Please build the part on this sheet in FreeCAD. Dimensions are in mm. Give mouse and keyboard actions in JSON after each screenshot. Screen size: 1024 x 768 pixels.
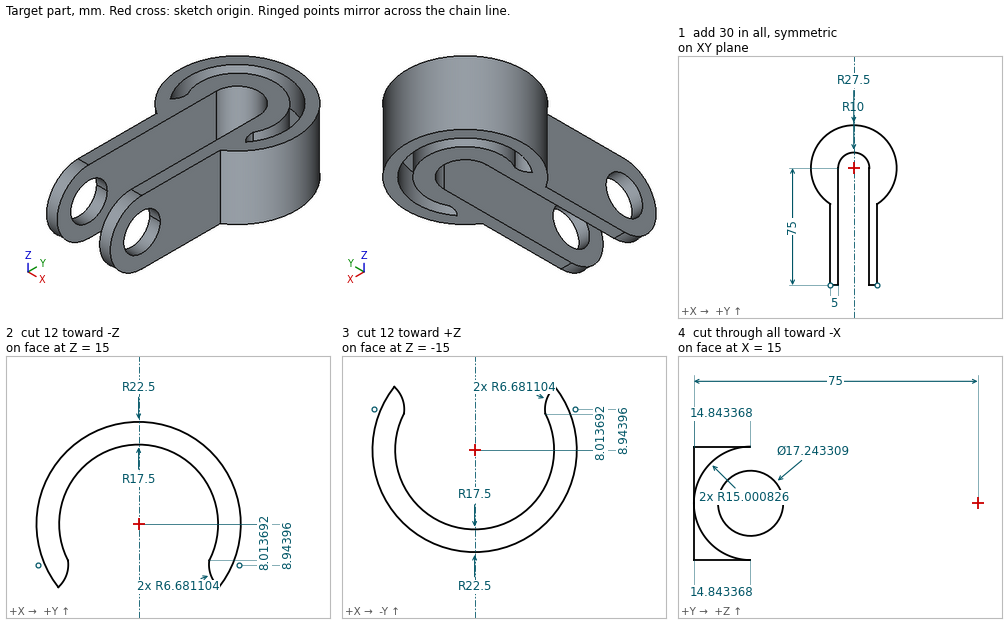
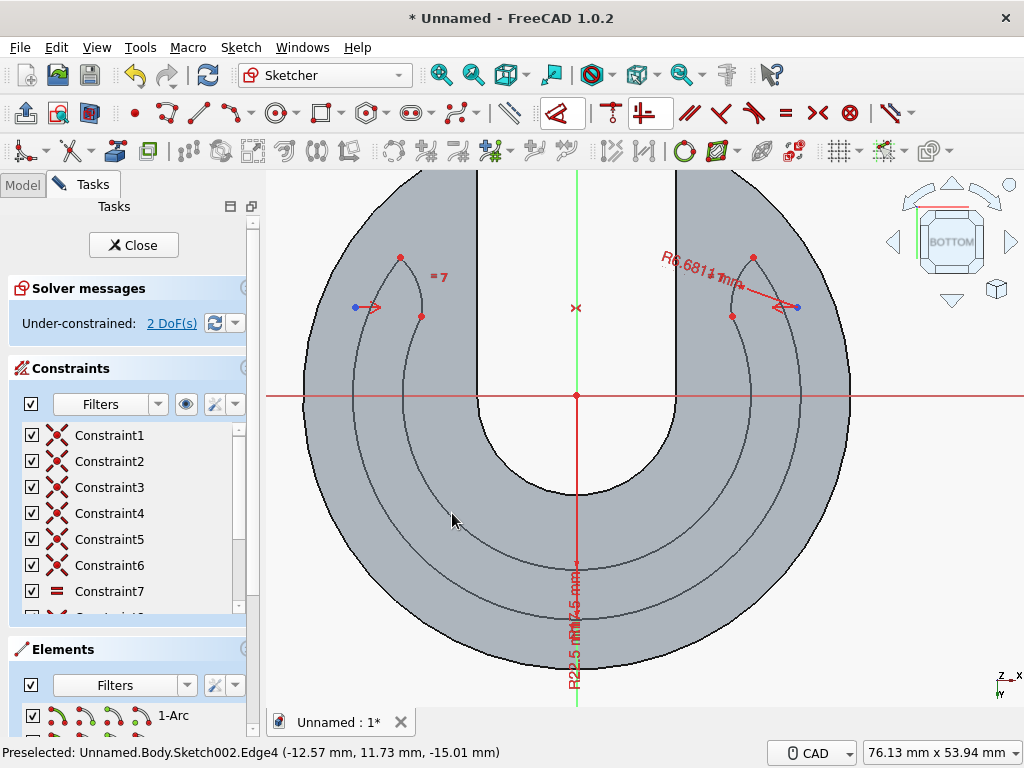
{"action": "left_click", "coordinate": [798, 307]}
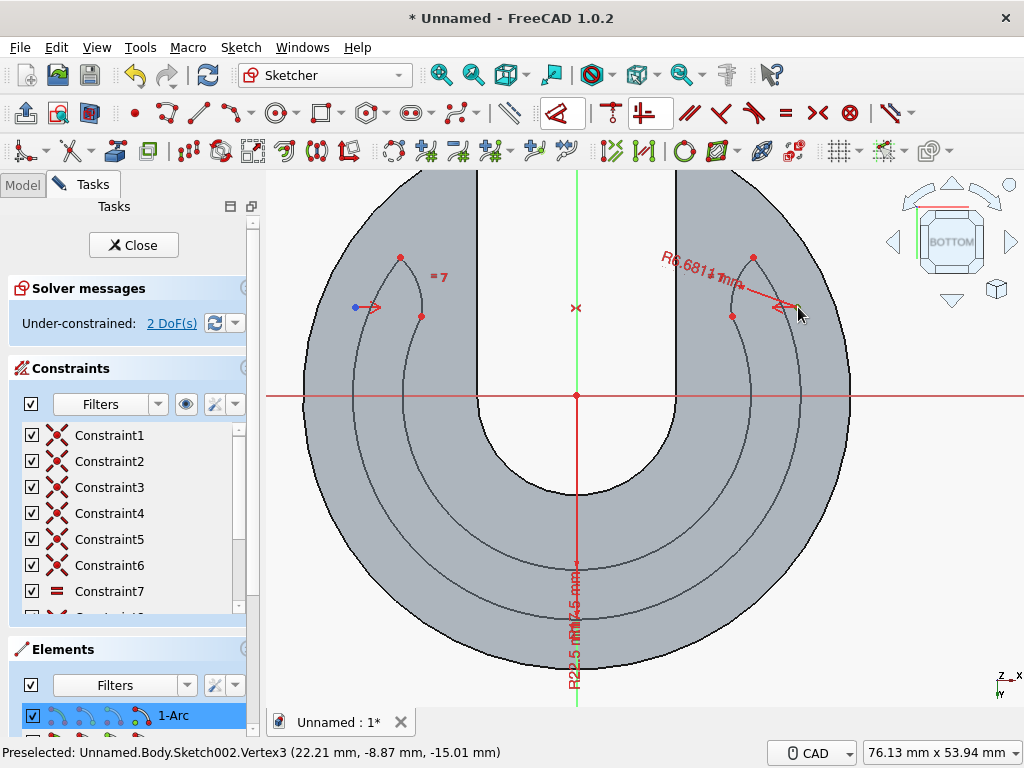
{"action": "key", "text": "i"}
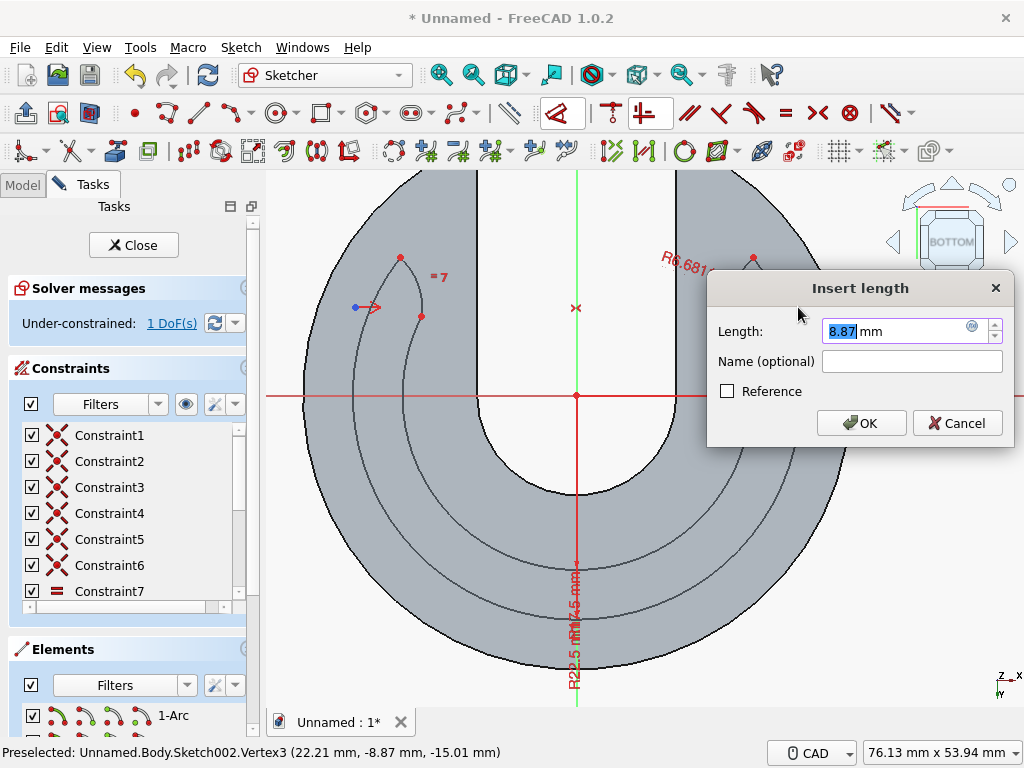
{"action": "type", "text": "8.94396"}
{"action": "key", "text": "Return"}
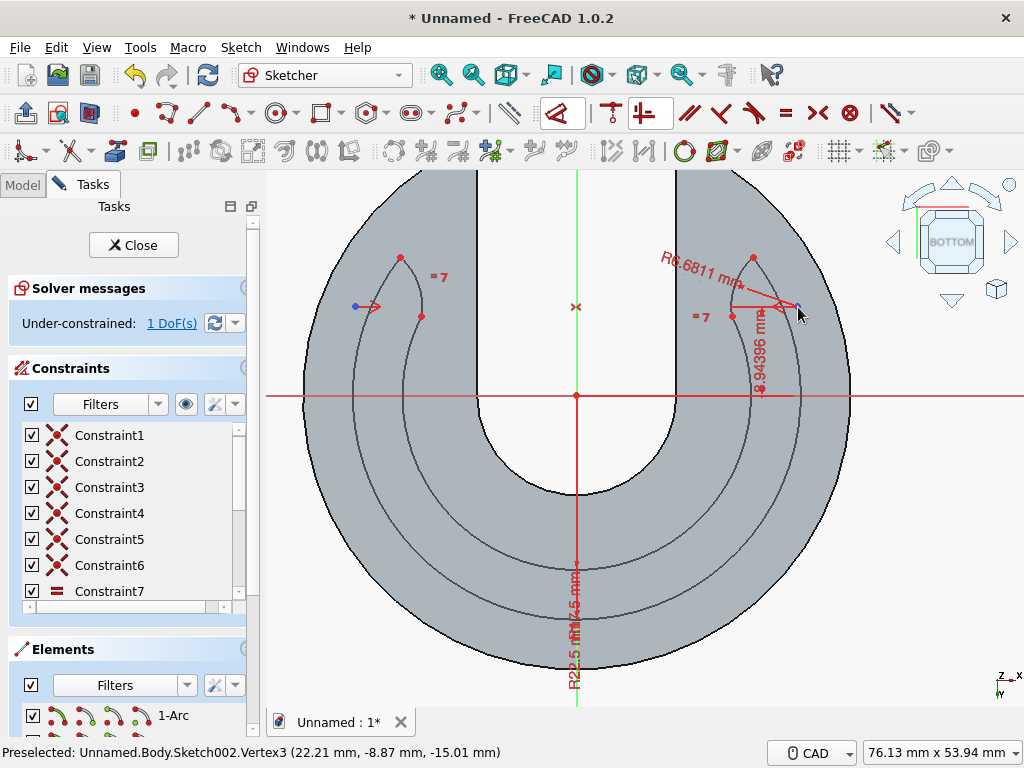
{"action": "left_click", "coordinate": [732, 317]}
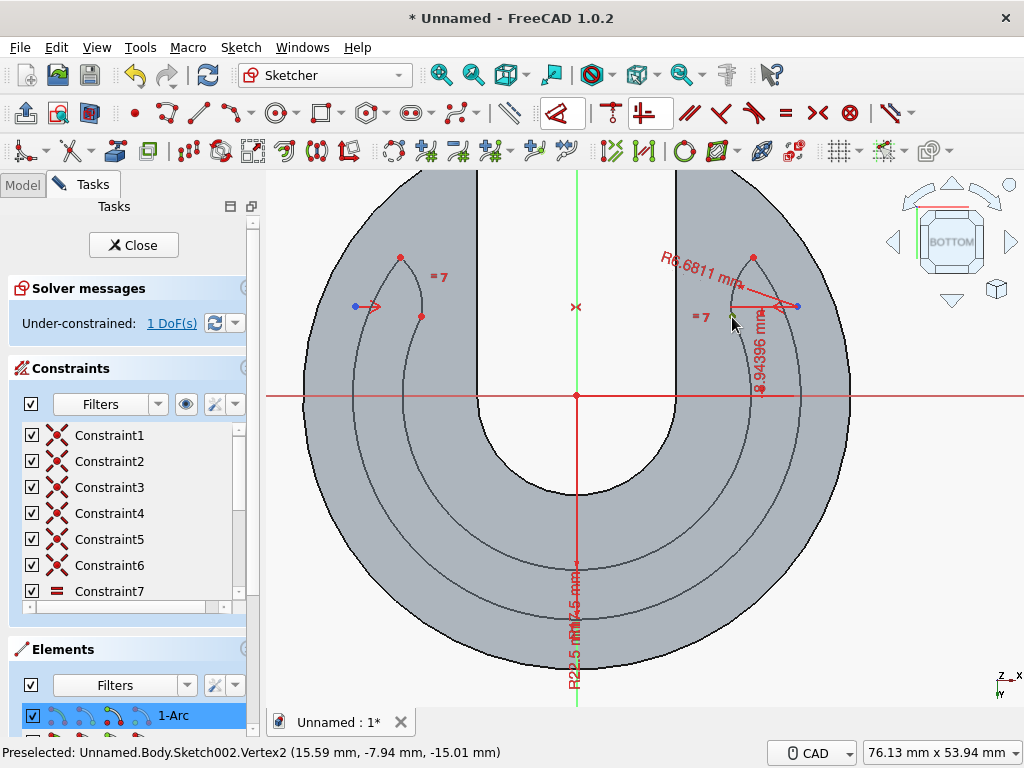
{"action": "key", "text": "i"}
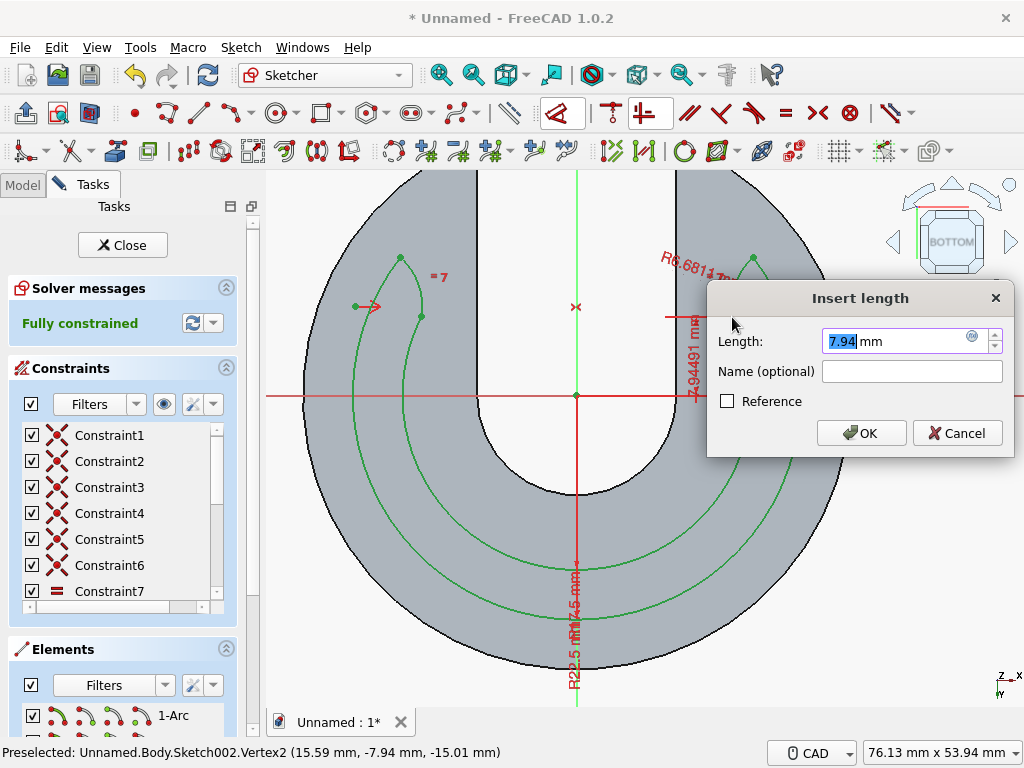
{"action": "type", "text": "8.013692"}
{"action": "key", "text": "Return"}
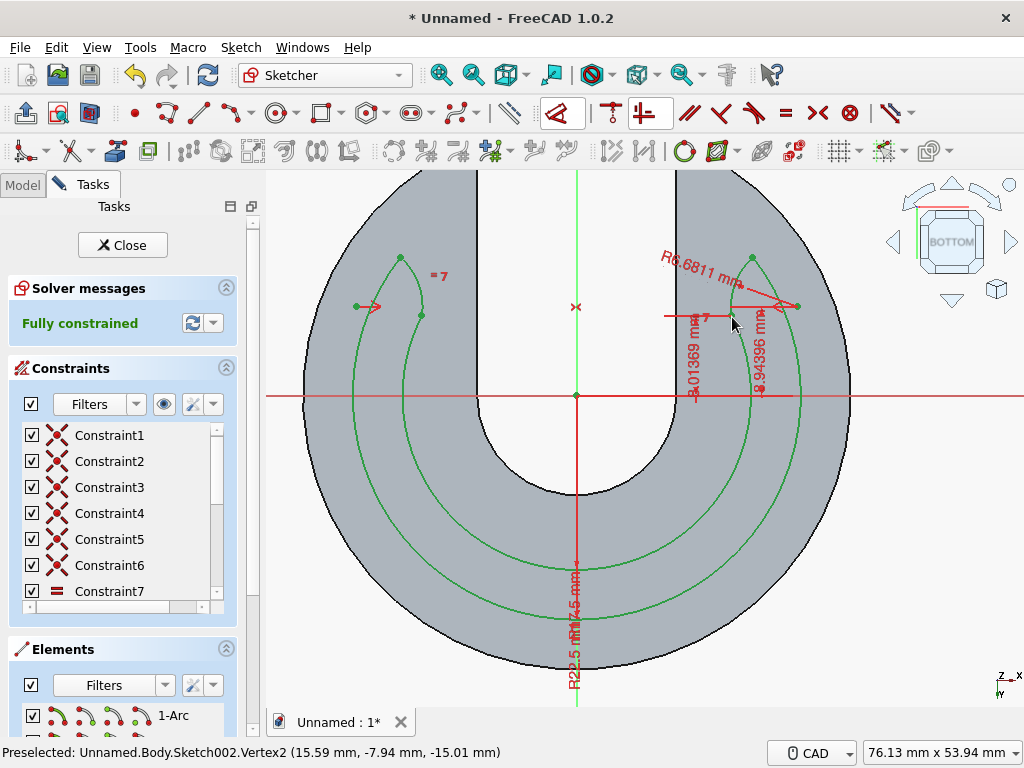
{"action": "left_click", "coordinate": [123, 245]}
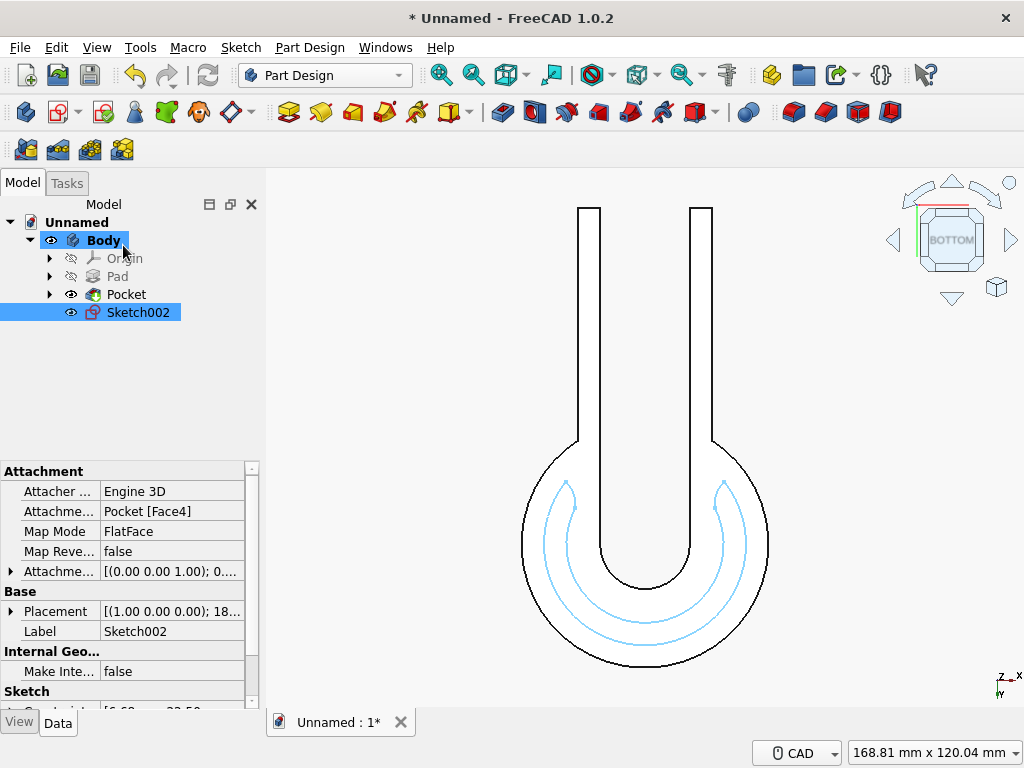
{"action": "left_click", "coordinate": [504, 112]}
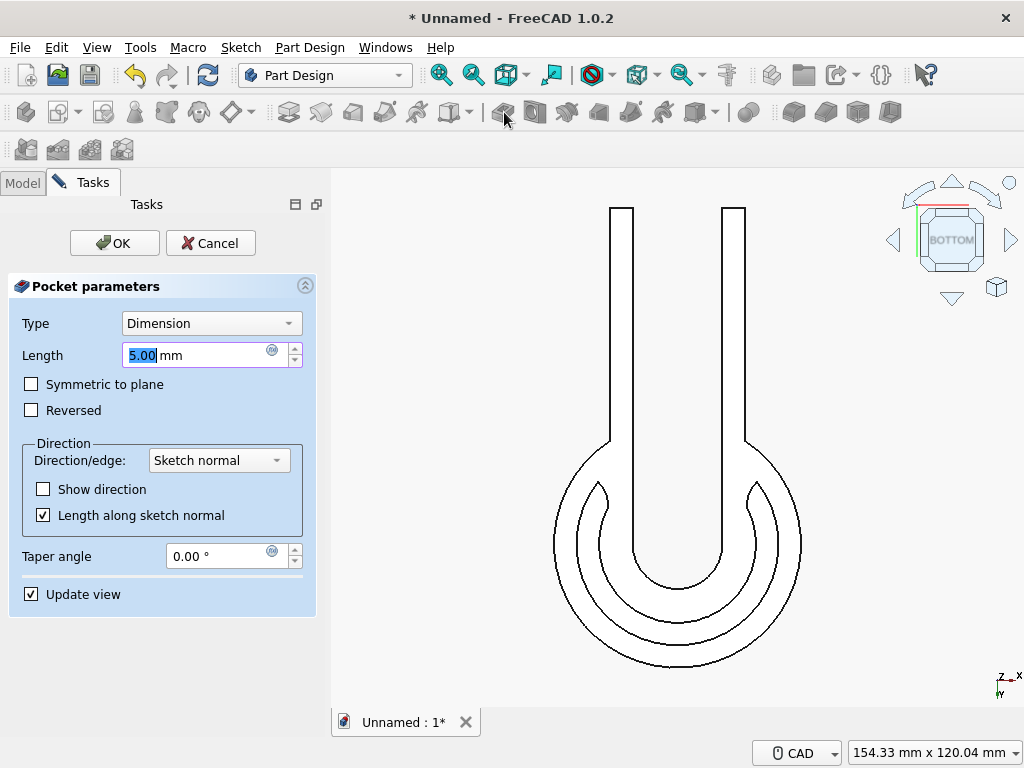
{"action": "type", "text": "12"}
{"action": "key", "text": "Tab"}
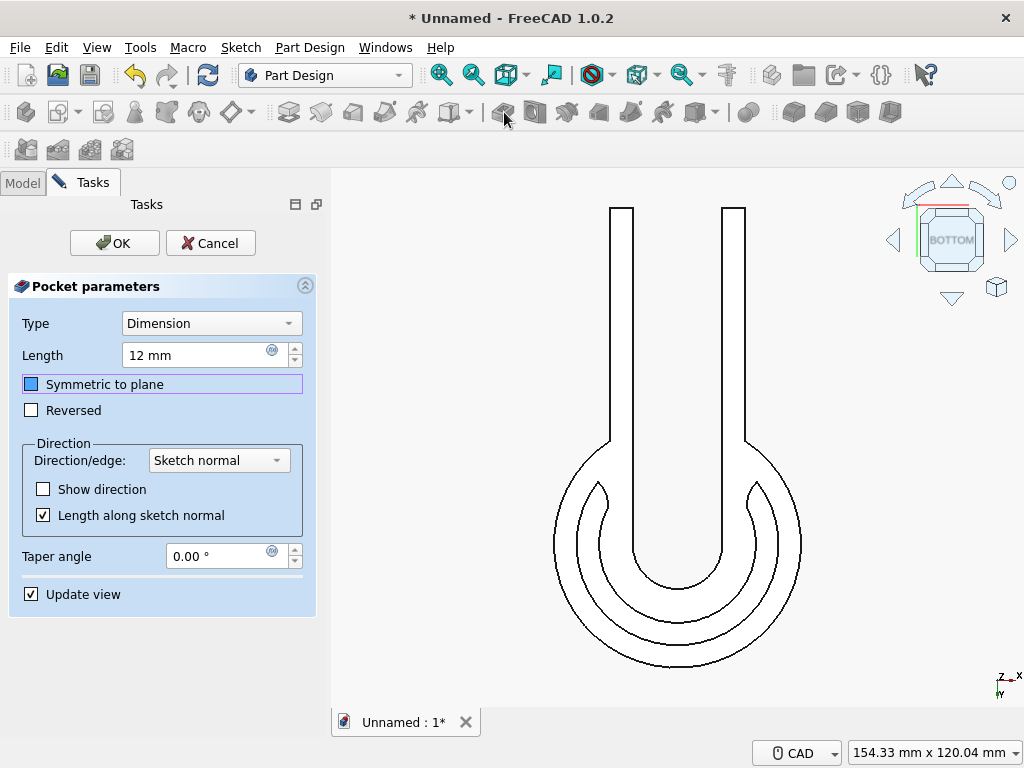
{"action": "left_click", "coordinate": [115, 243]}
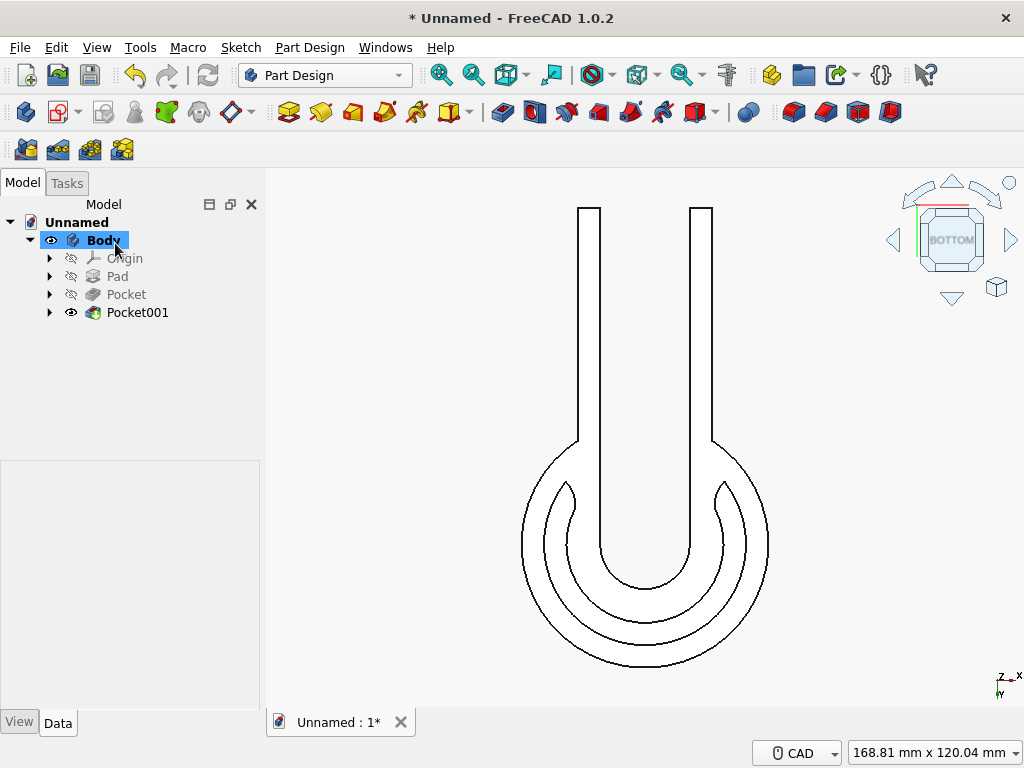
{"action": "key", "text": "0"}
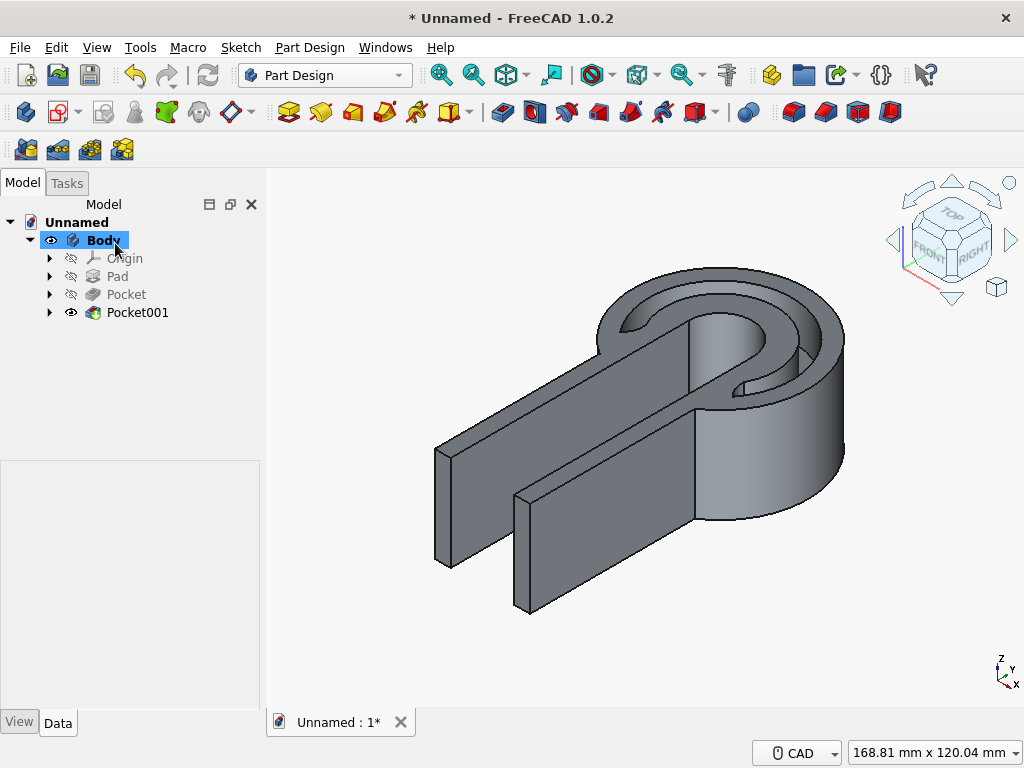
{"action": "left_click", "coordinate": [636, 497]}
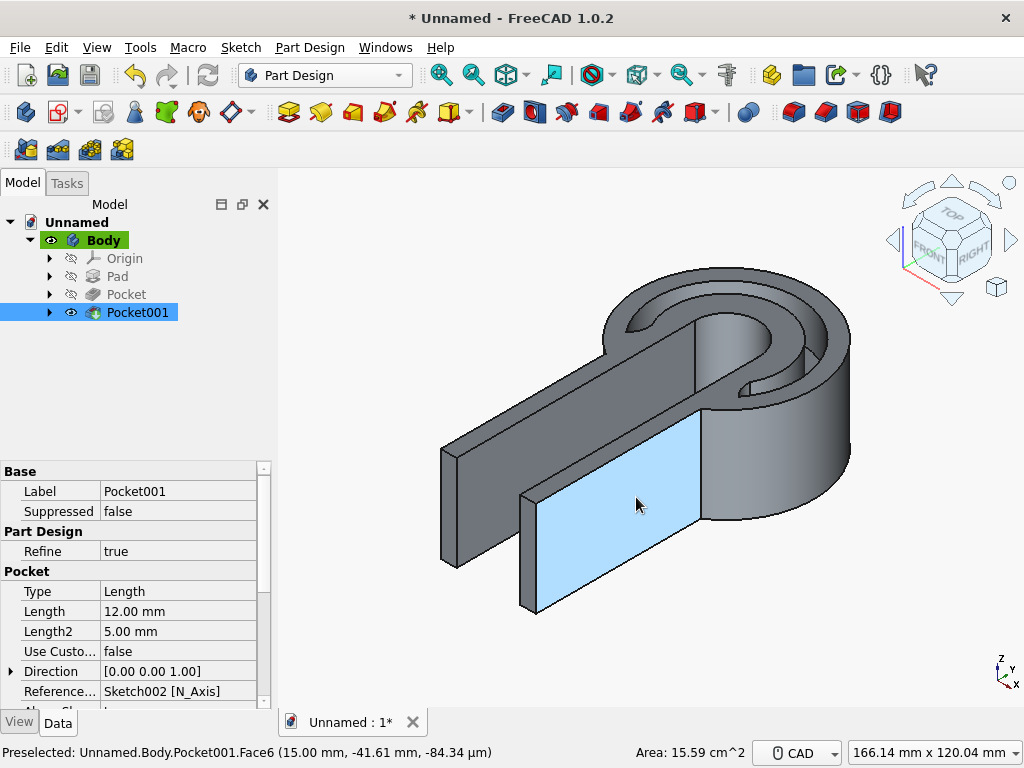
{"action": "left_click", "coordinate": [58, 112]}